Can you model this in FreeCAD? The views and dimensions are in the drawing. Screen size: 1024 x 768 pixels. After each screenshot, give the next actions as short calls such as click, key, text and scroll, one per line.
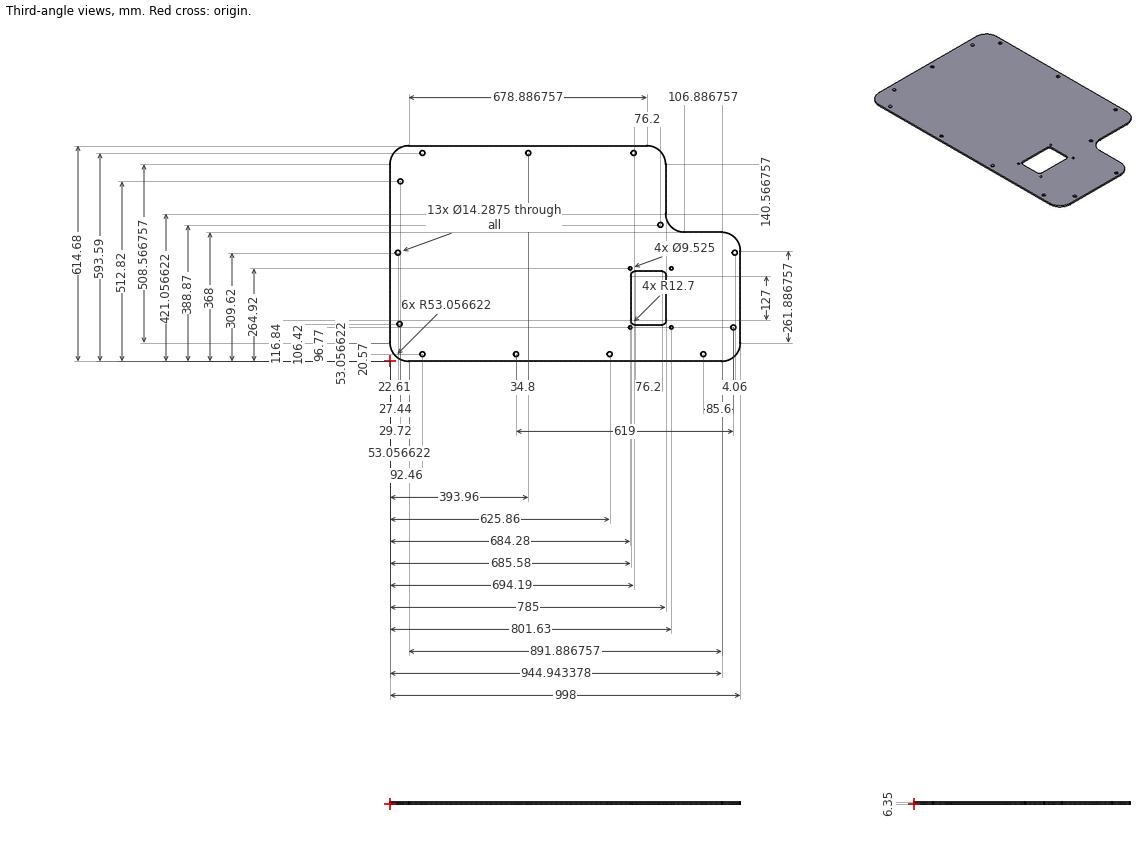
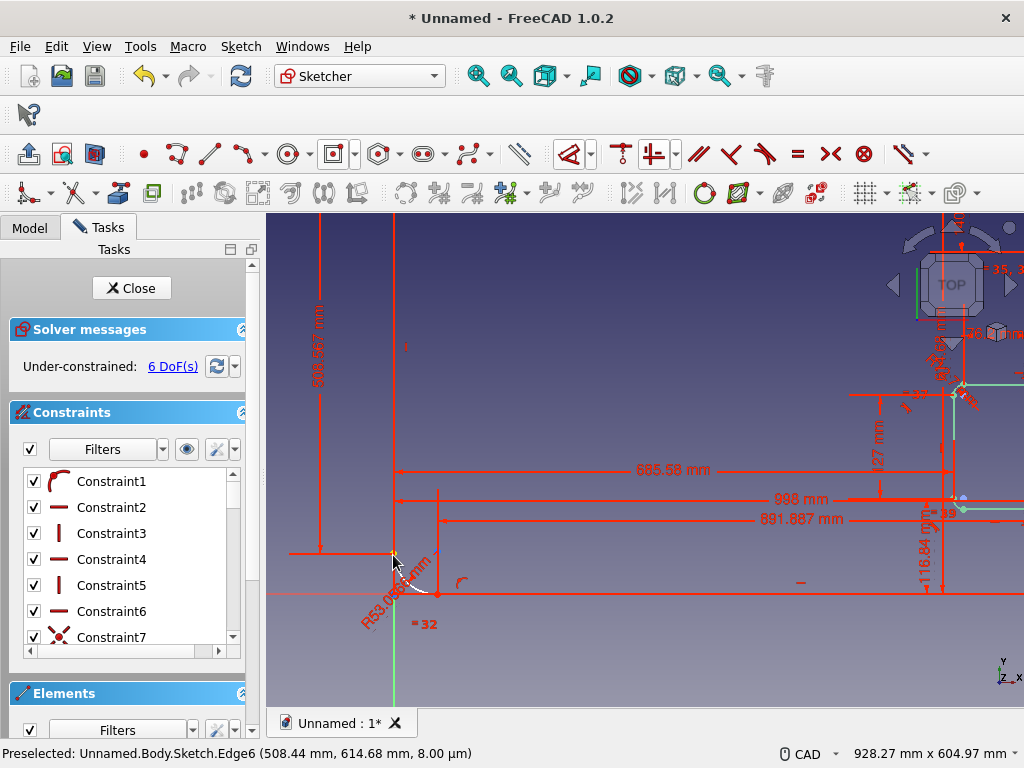
click(394, 554)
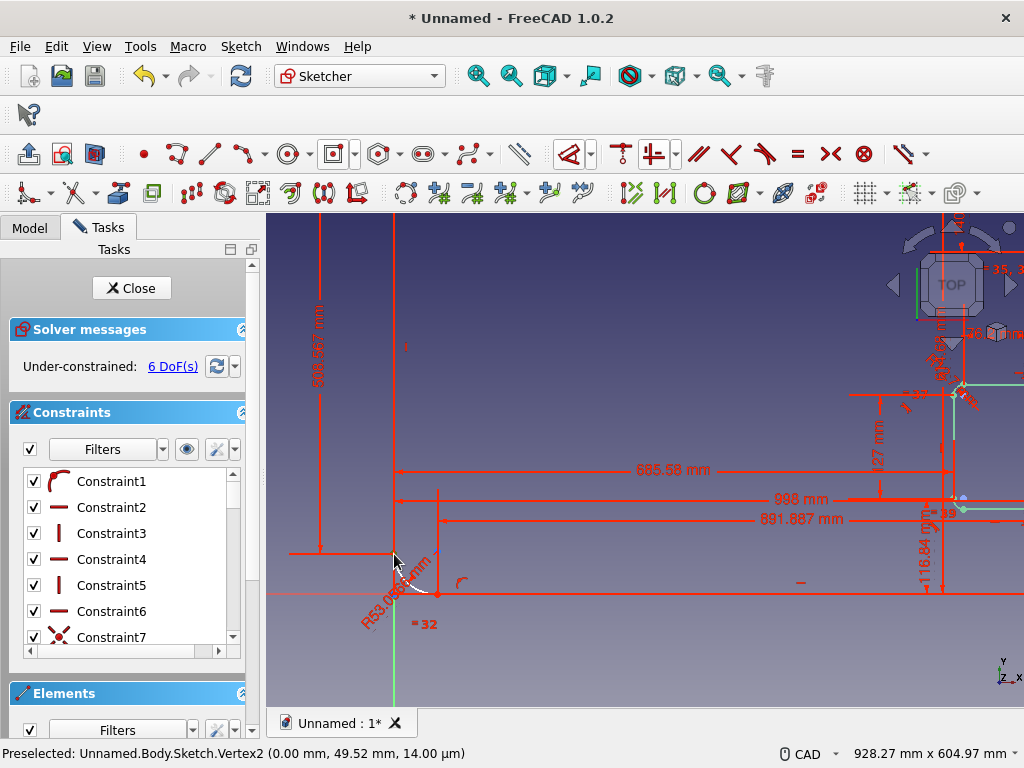
click(590, 154)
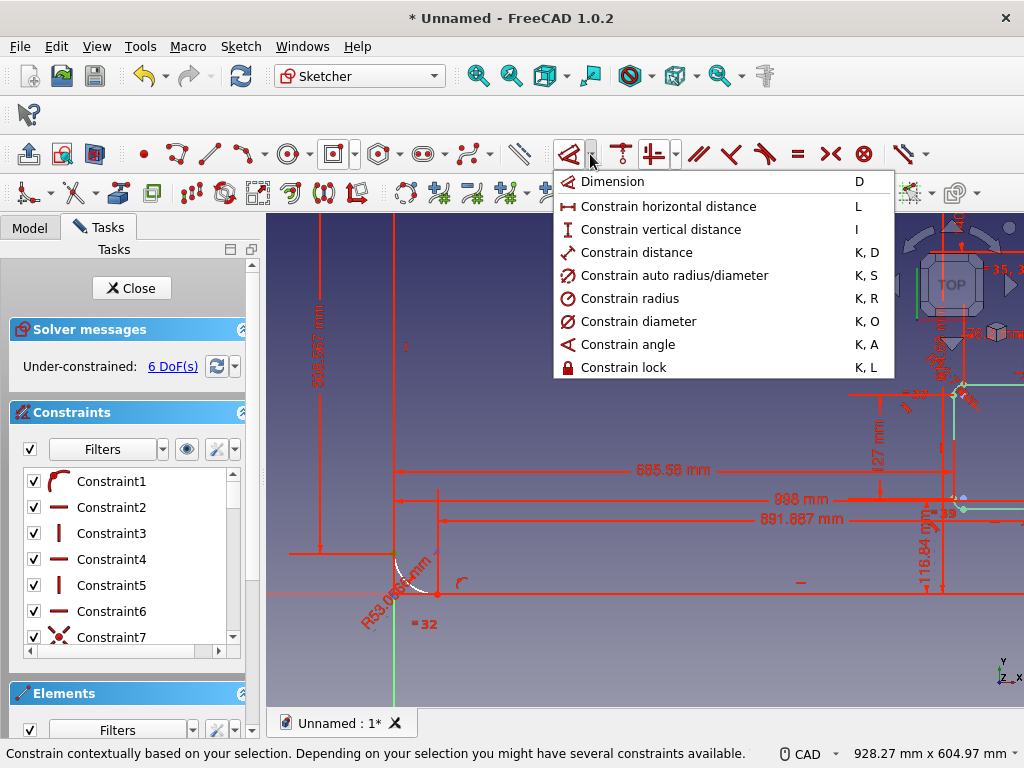
click(724, 230)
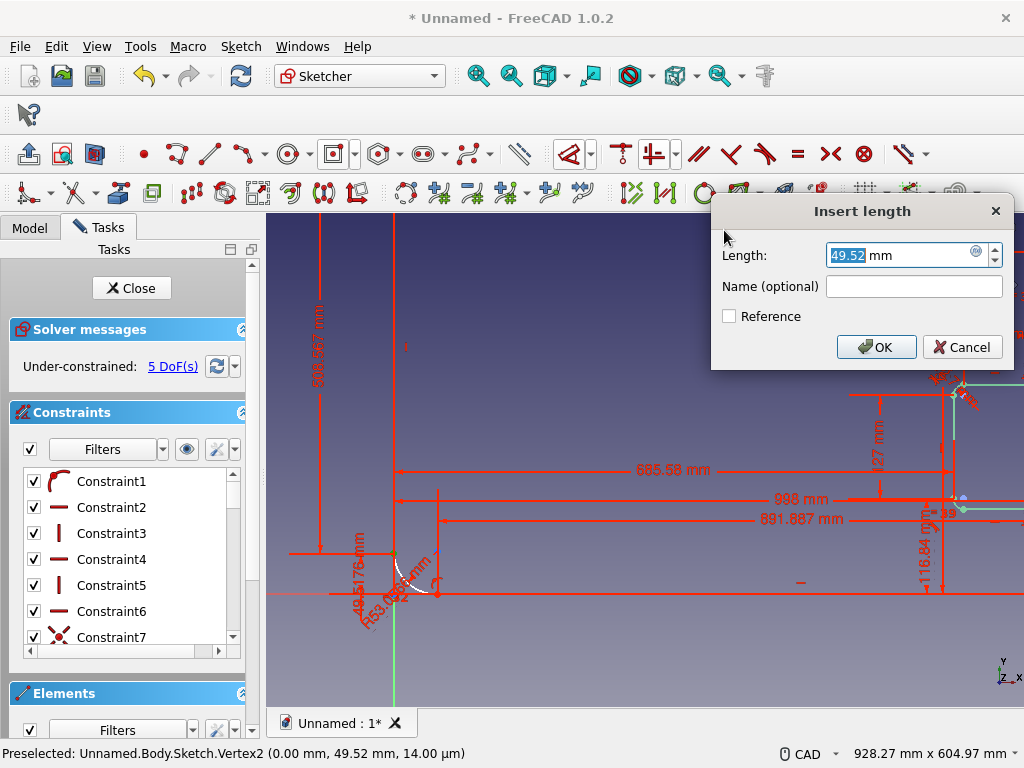
text(53.056622)
key(Return)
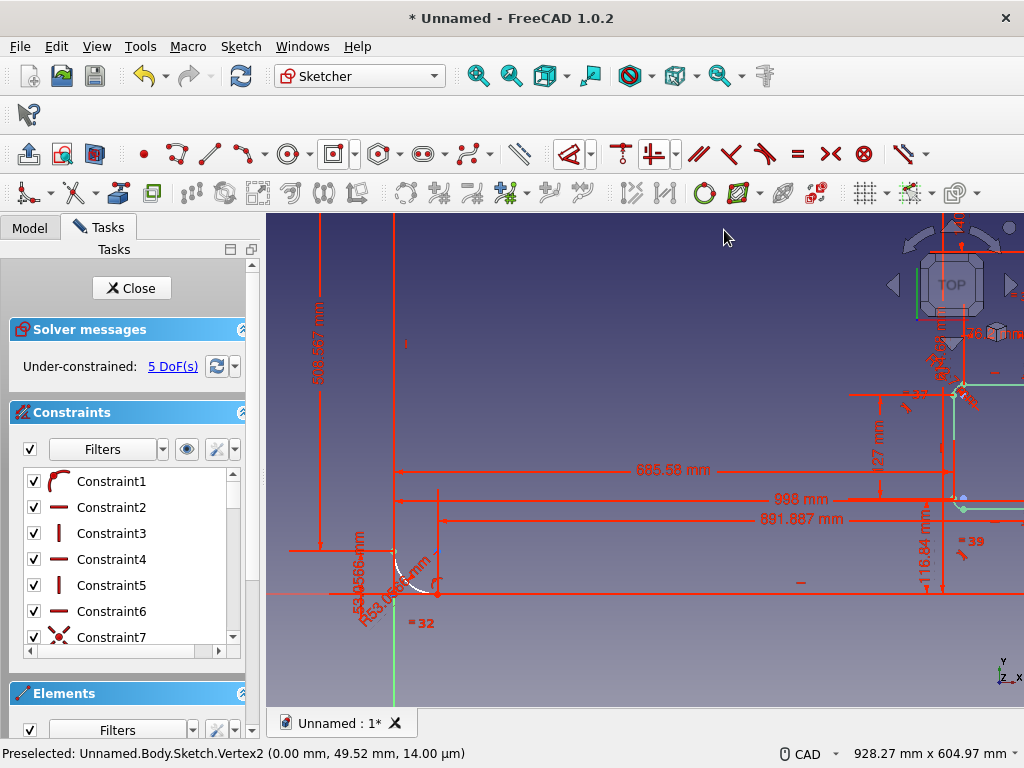
click(438, 594)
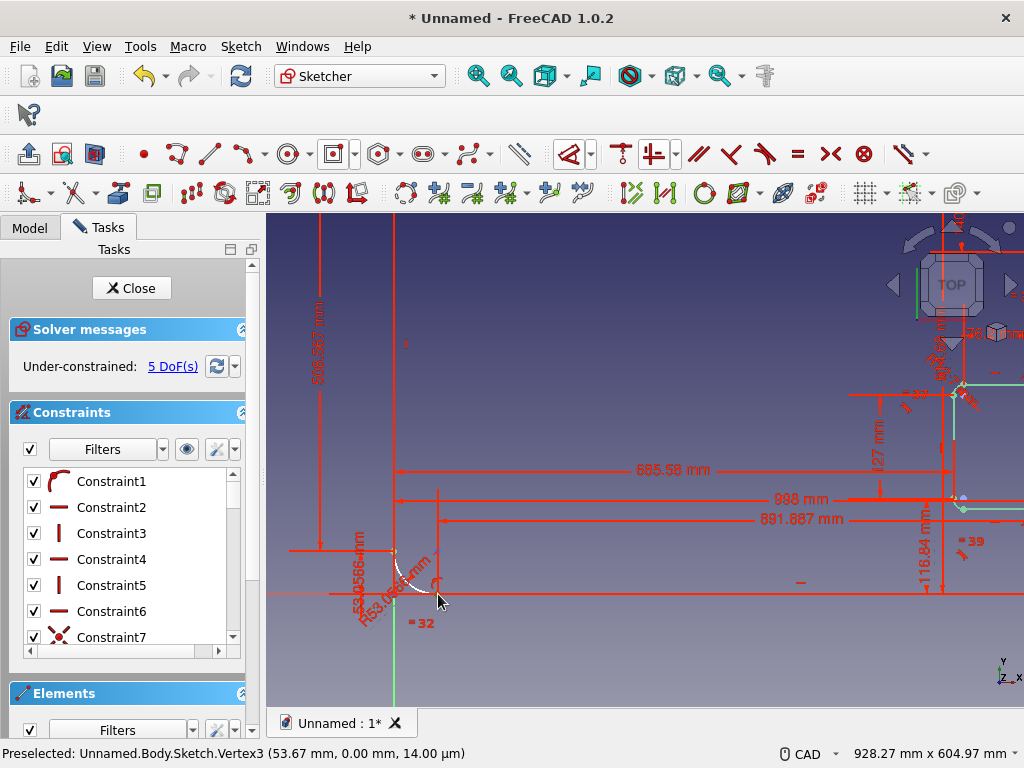
click(590, 154)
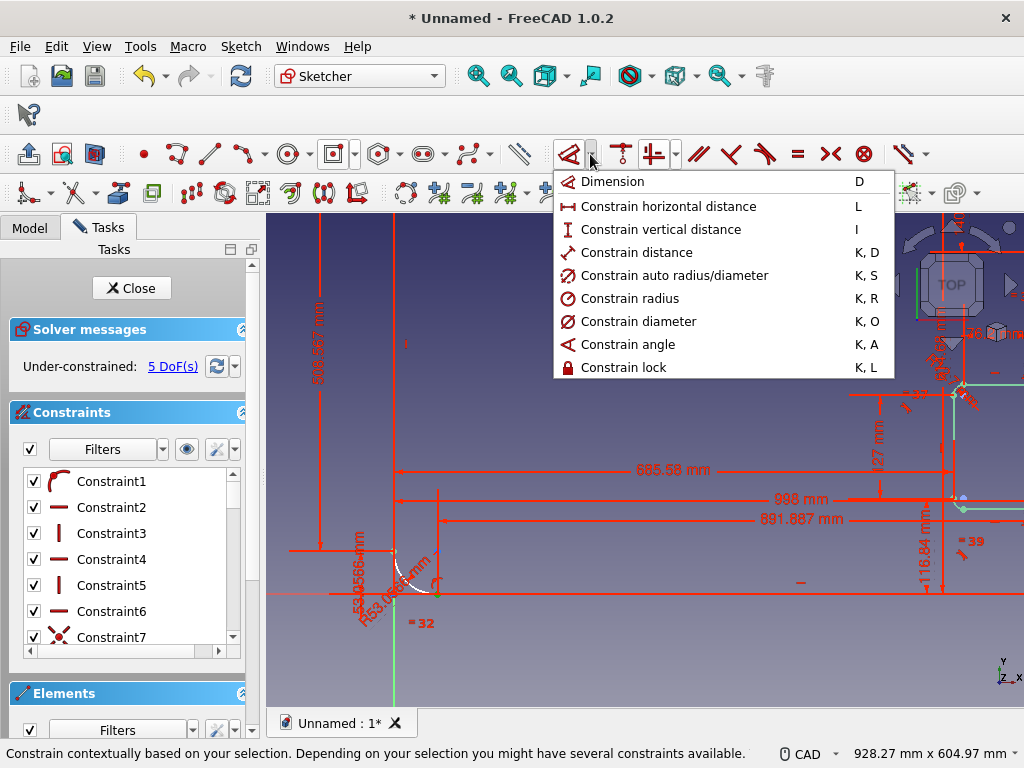
click(724, 206)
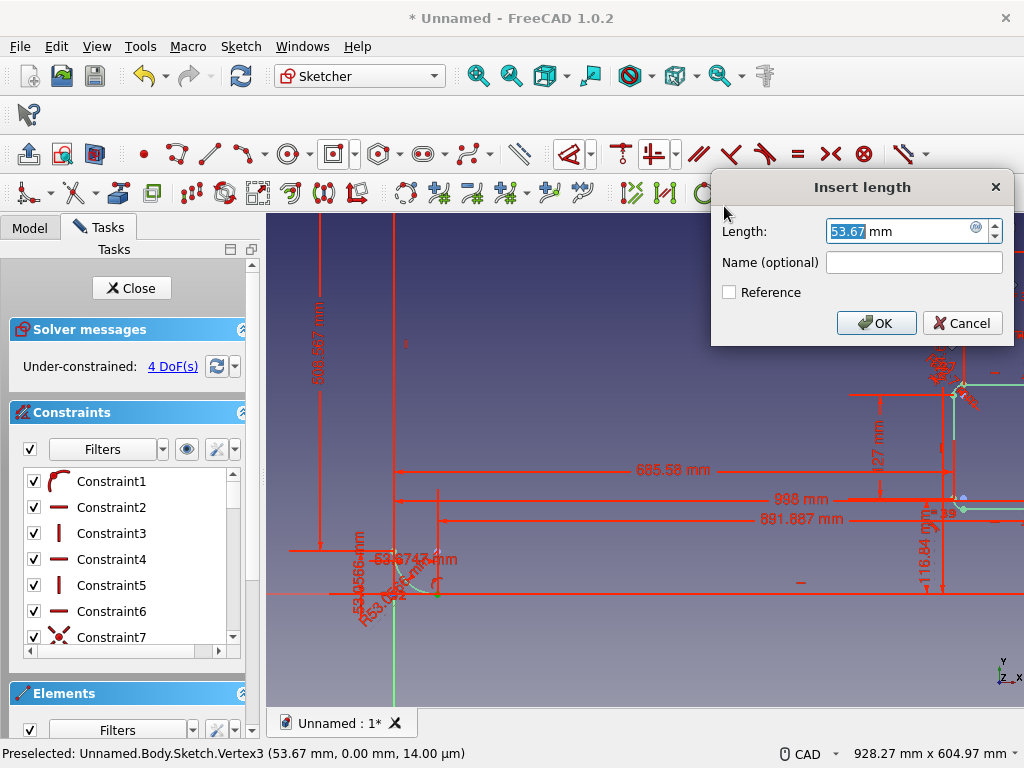
text(53.056622)
key(Return)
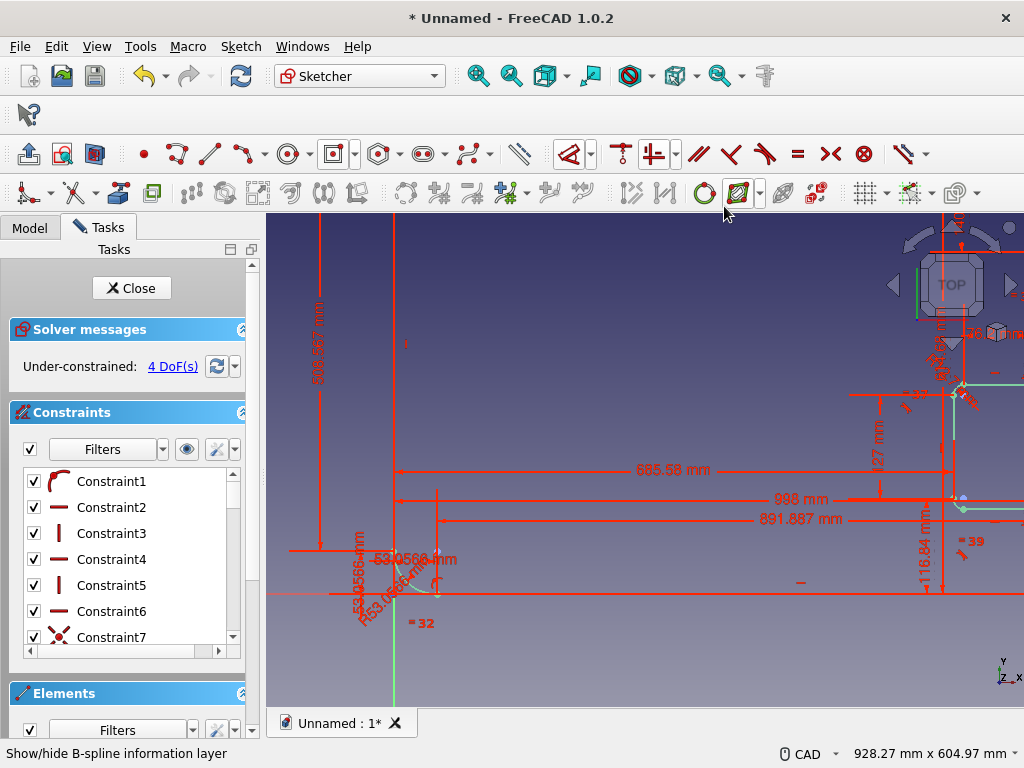
scroll(393, 555, down, 4)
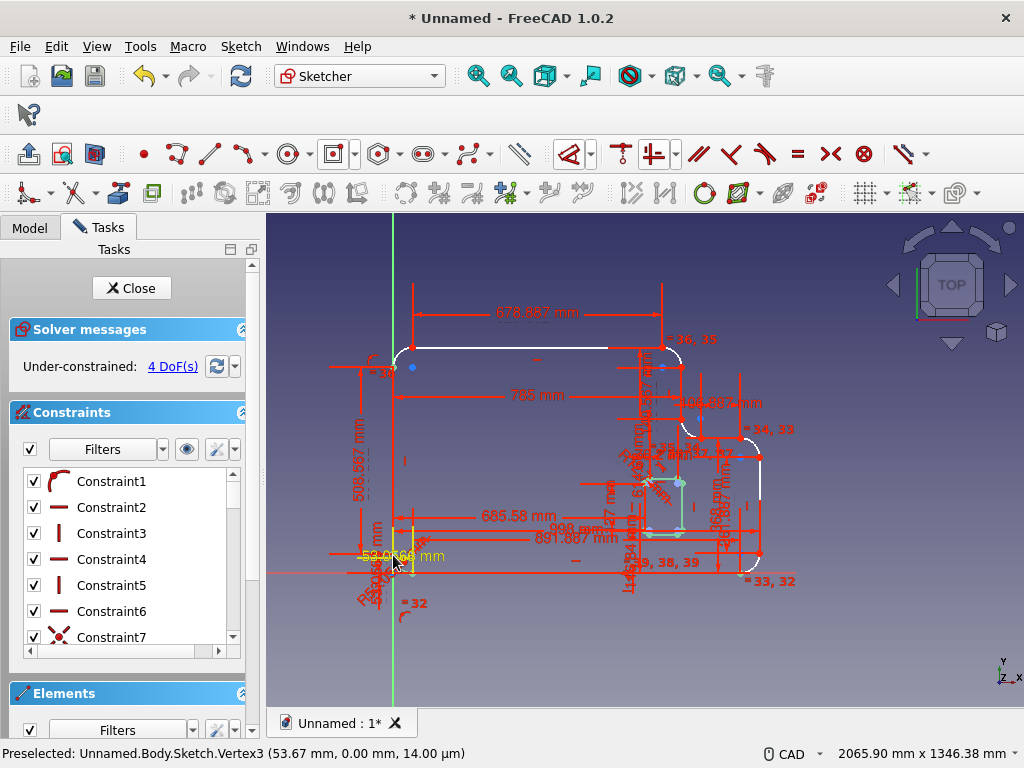
scroll(760, 553, up, 4)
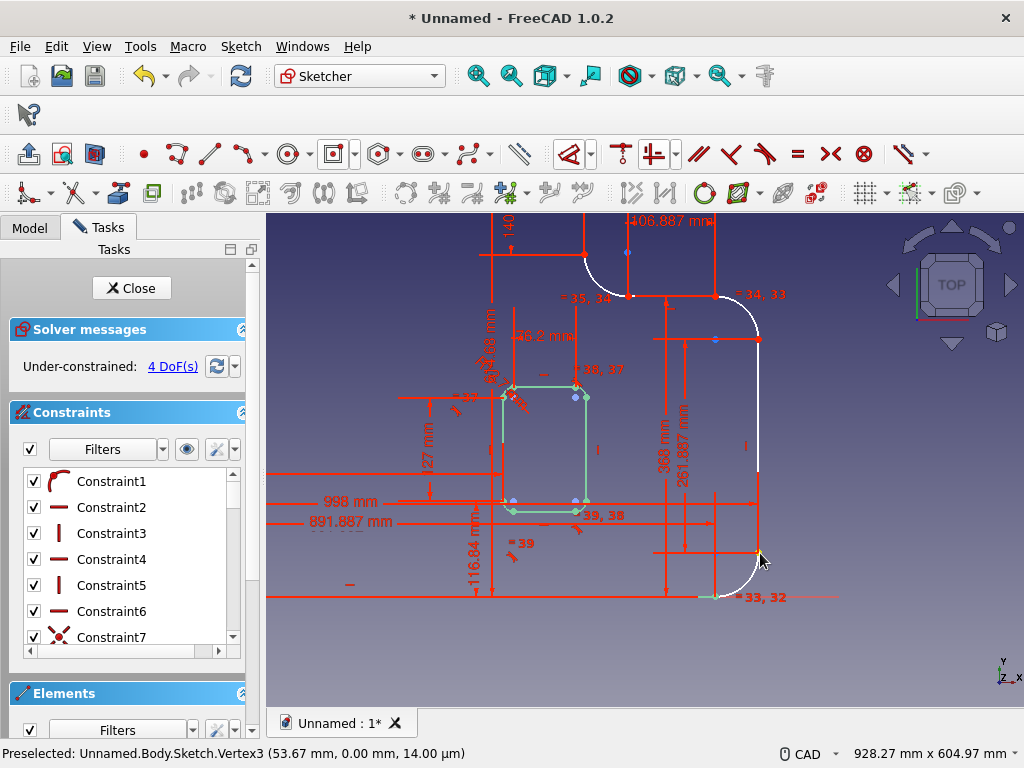
click(758, 553)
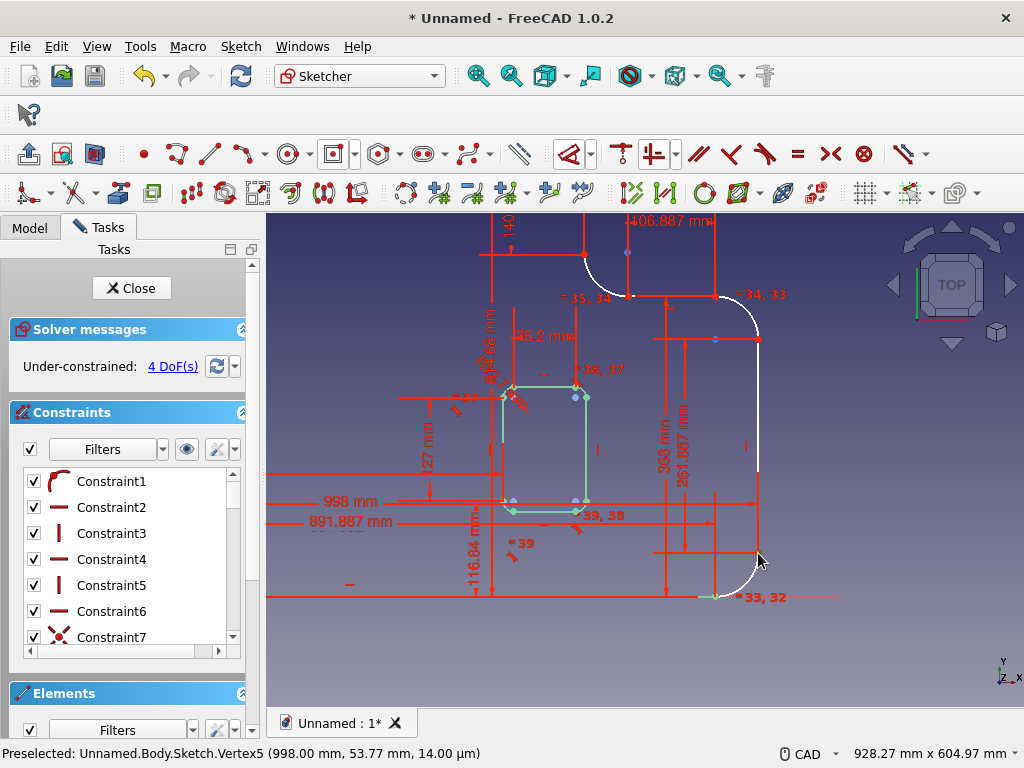
key(i)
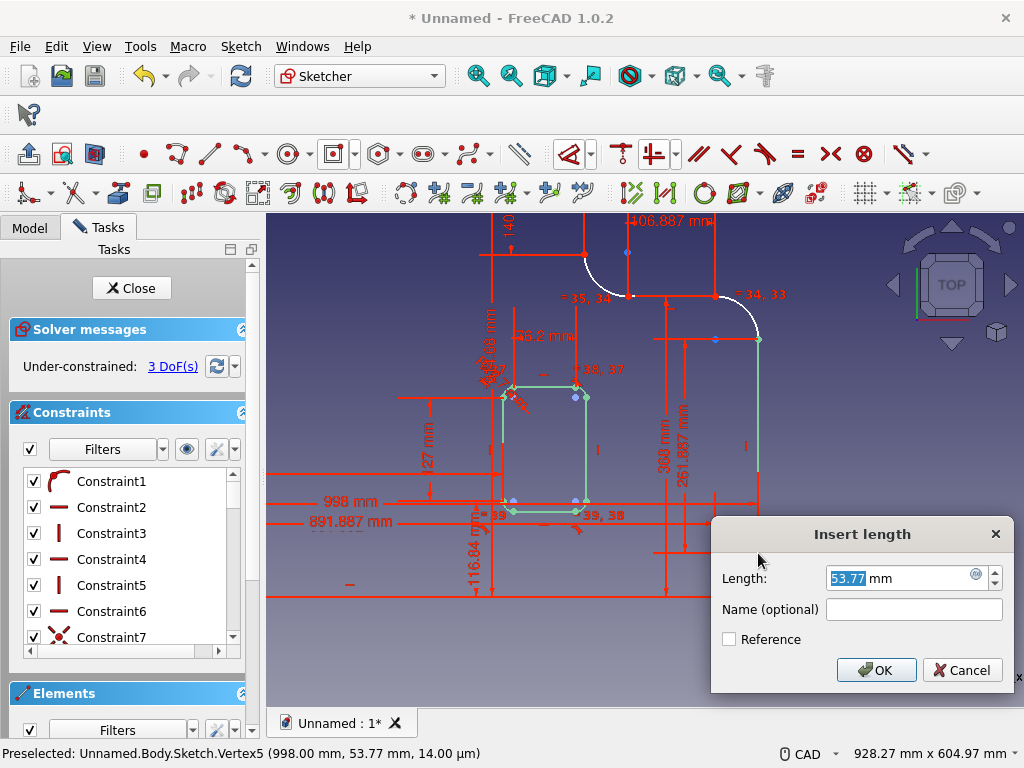
text(53.056622)
key(Return)